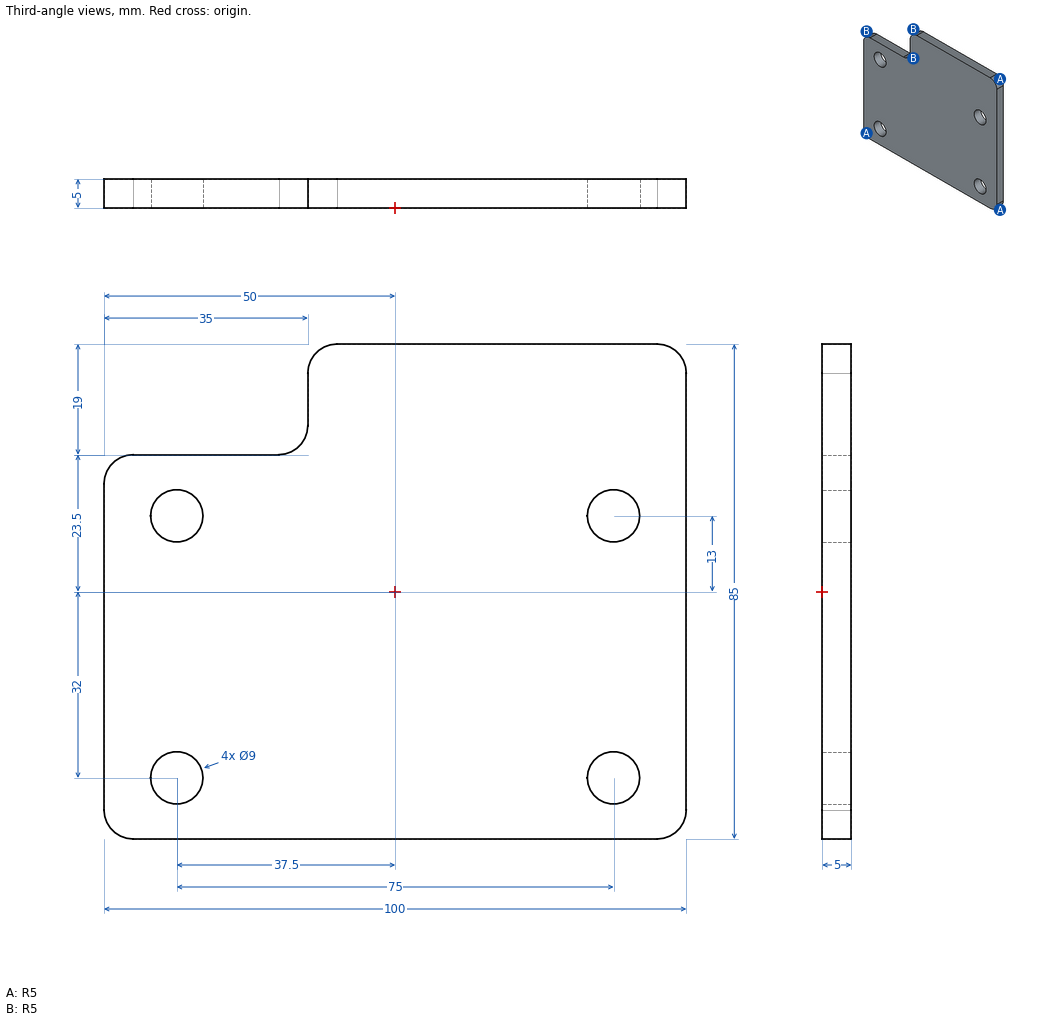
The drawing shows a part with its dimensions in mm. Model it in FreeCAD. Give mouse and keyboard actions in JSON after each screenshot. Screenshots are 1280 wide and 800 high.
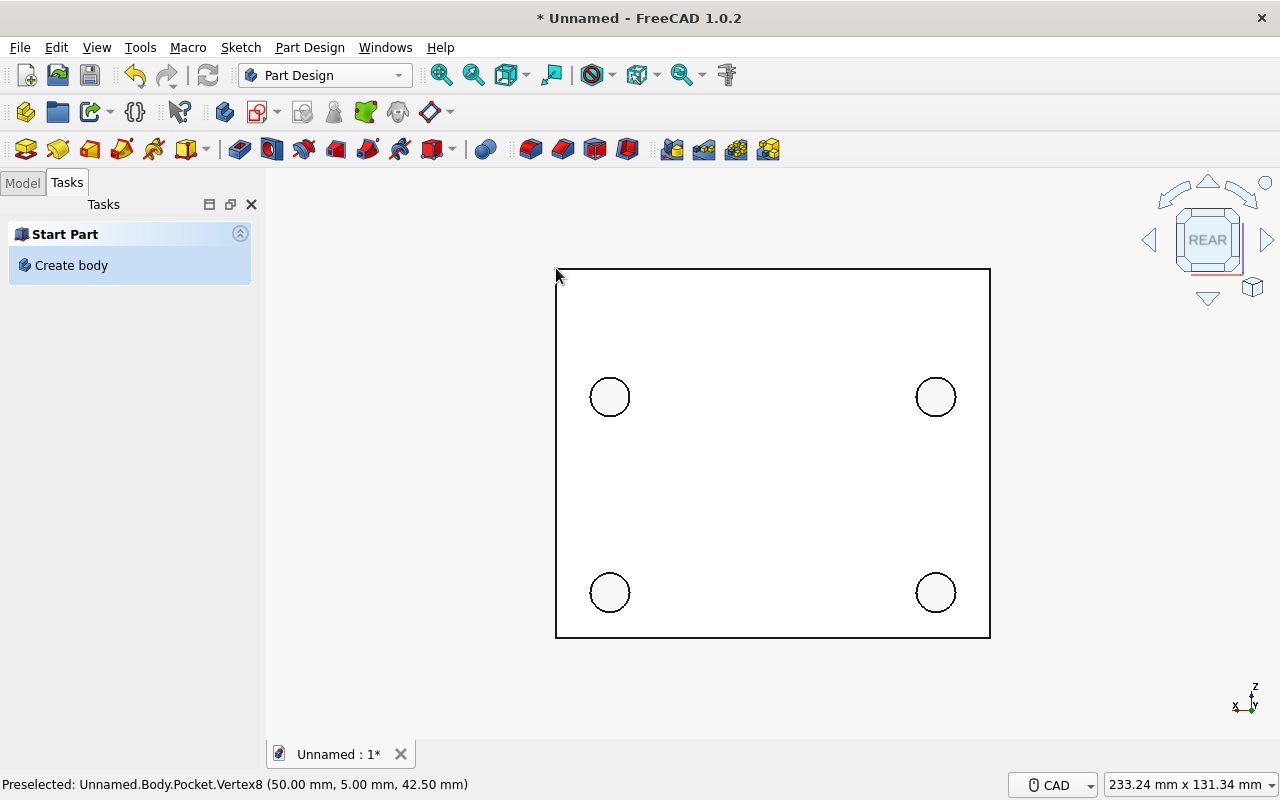
{"action": "key", "text": "0"}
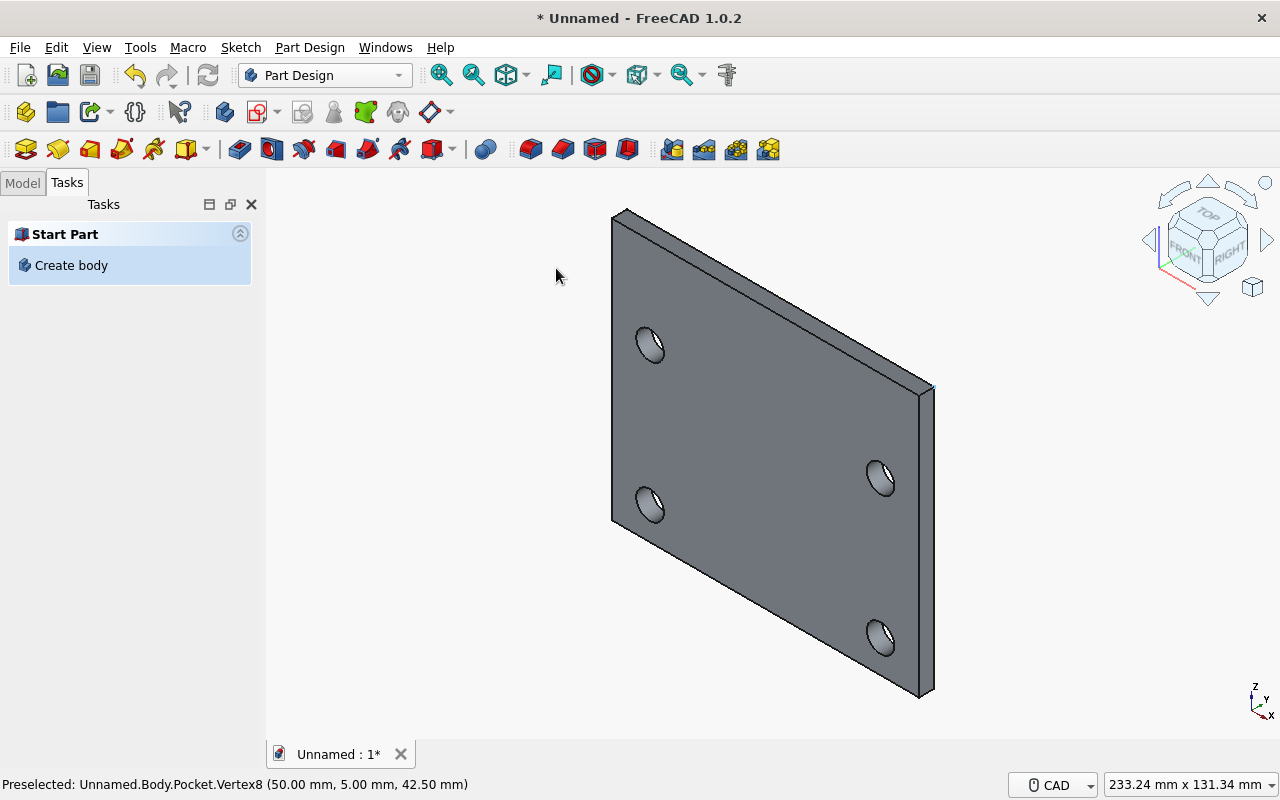
{"action": "left_click", "coordinate": [927, 390]}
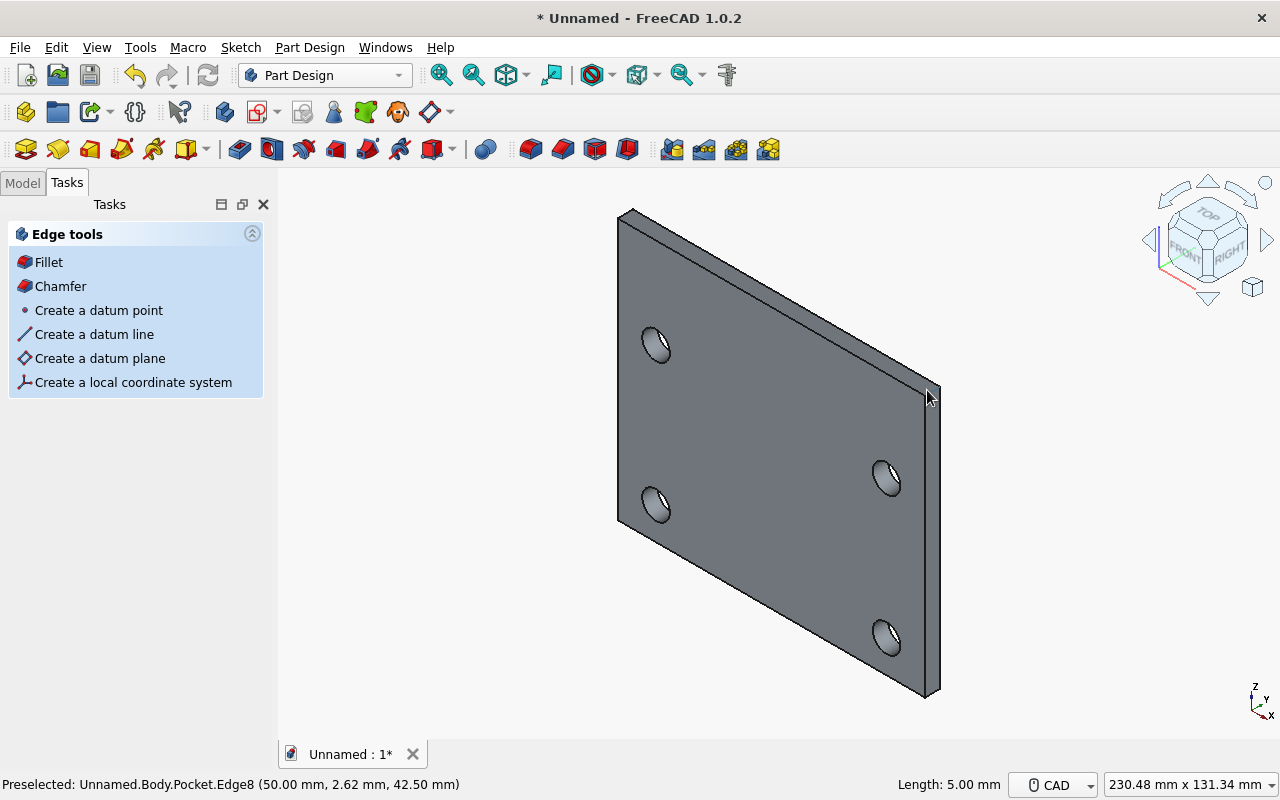
{"action": "scroll", "coordinate": [625, 515], "scroll_direction": "up", "scroll_amount": 4}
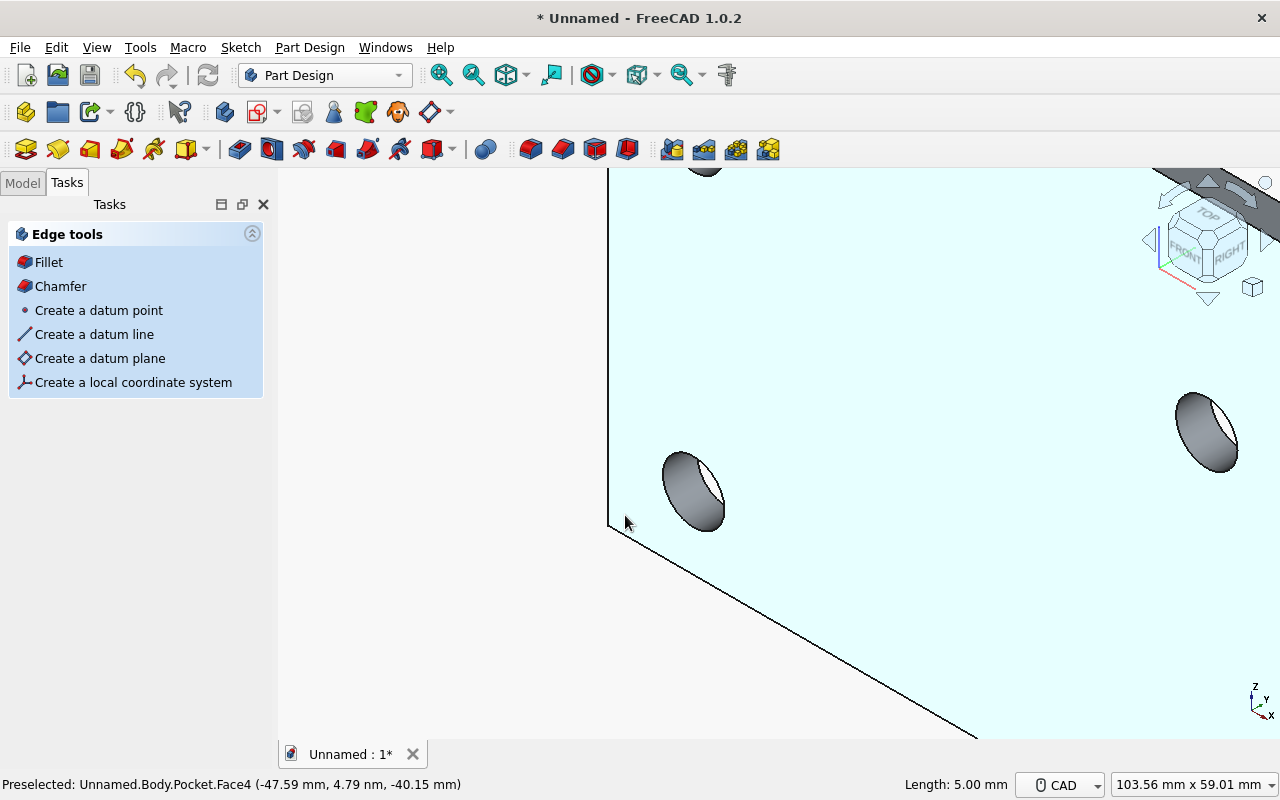
{"action": "left_click", "coordinate": [442, 76]}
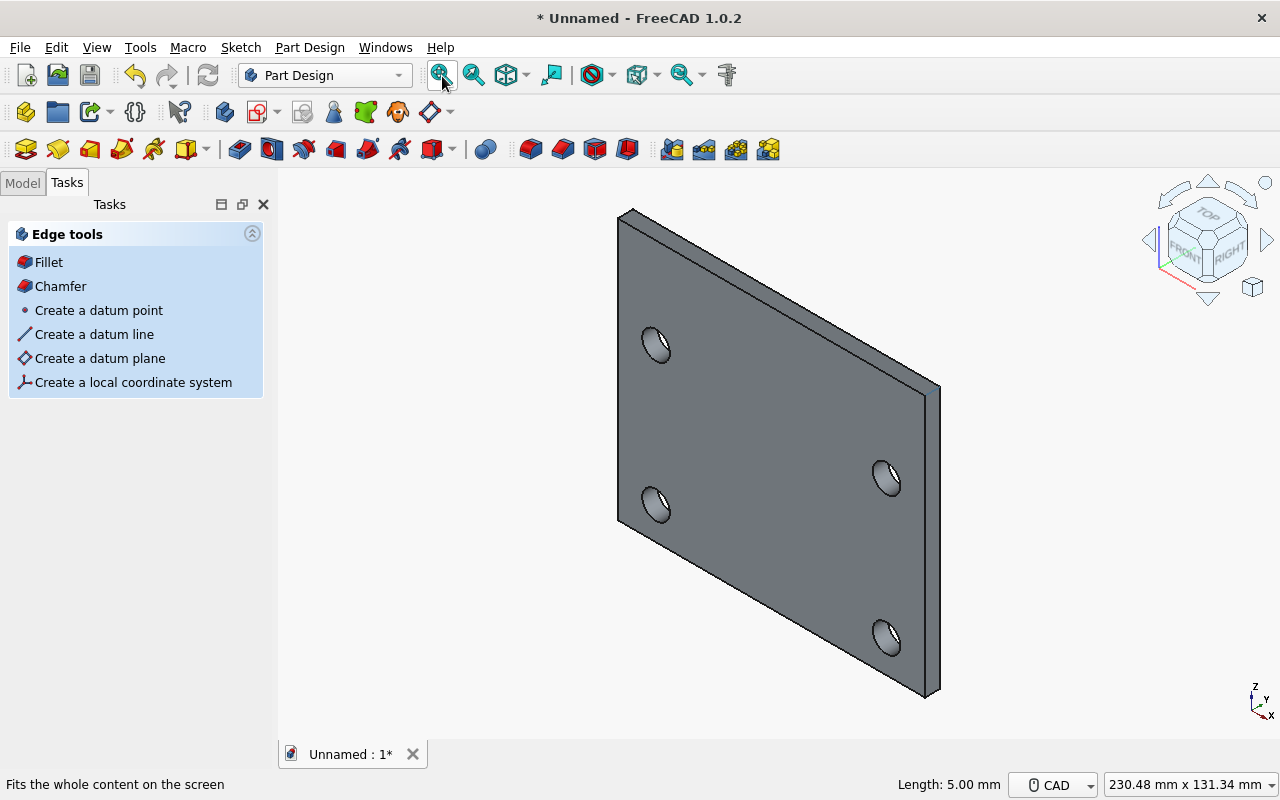
{"action": "key", "text": "2"}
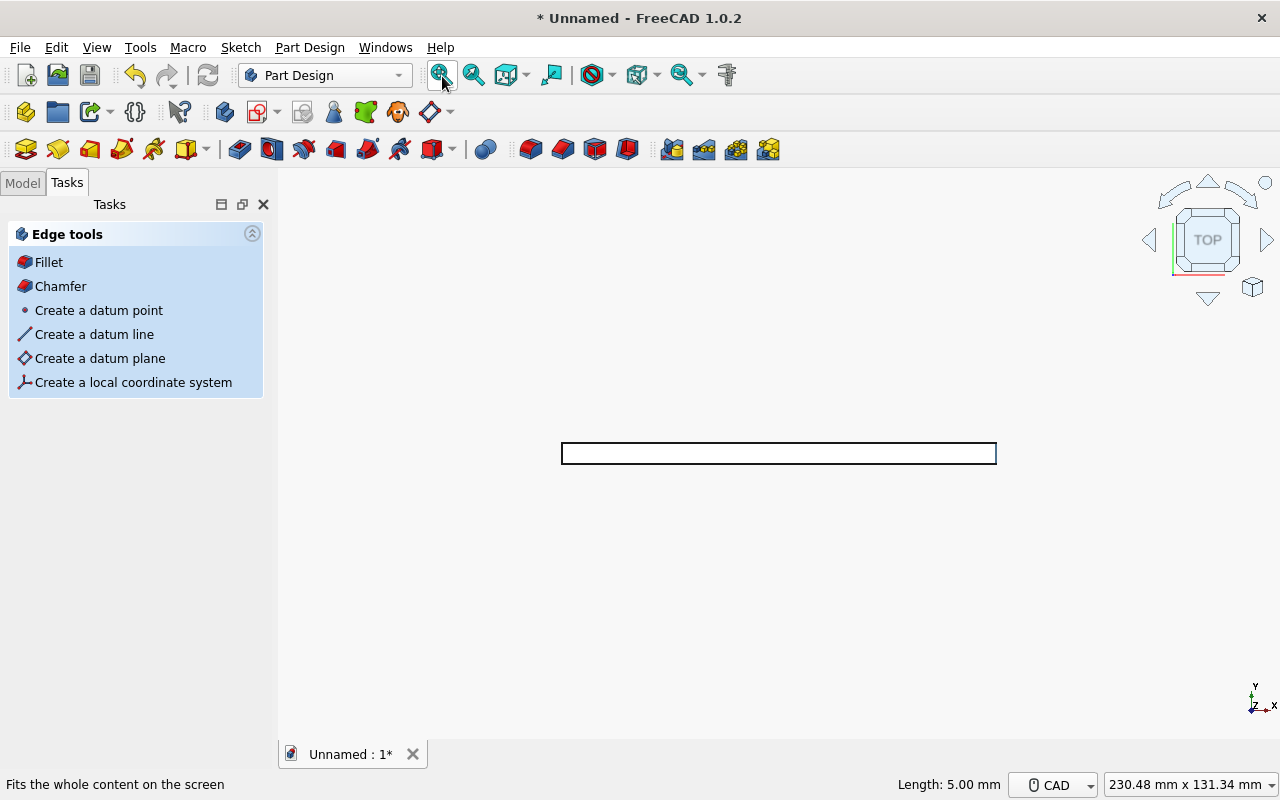
{"action": "left_click", "coordinate": [442, 76]}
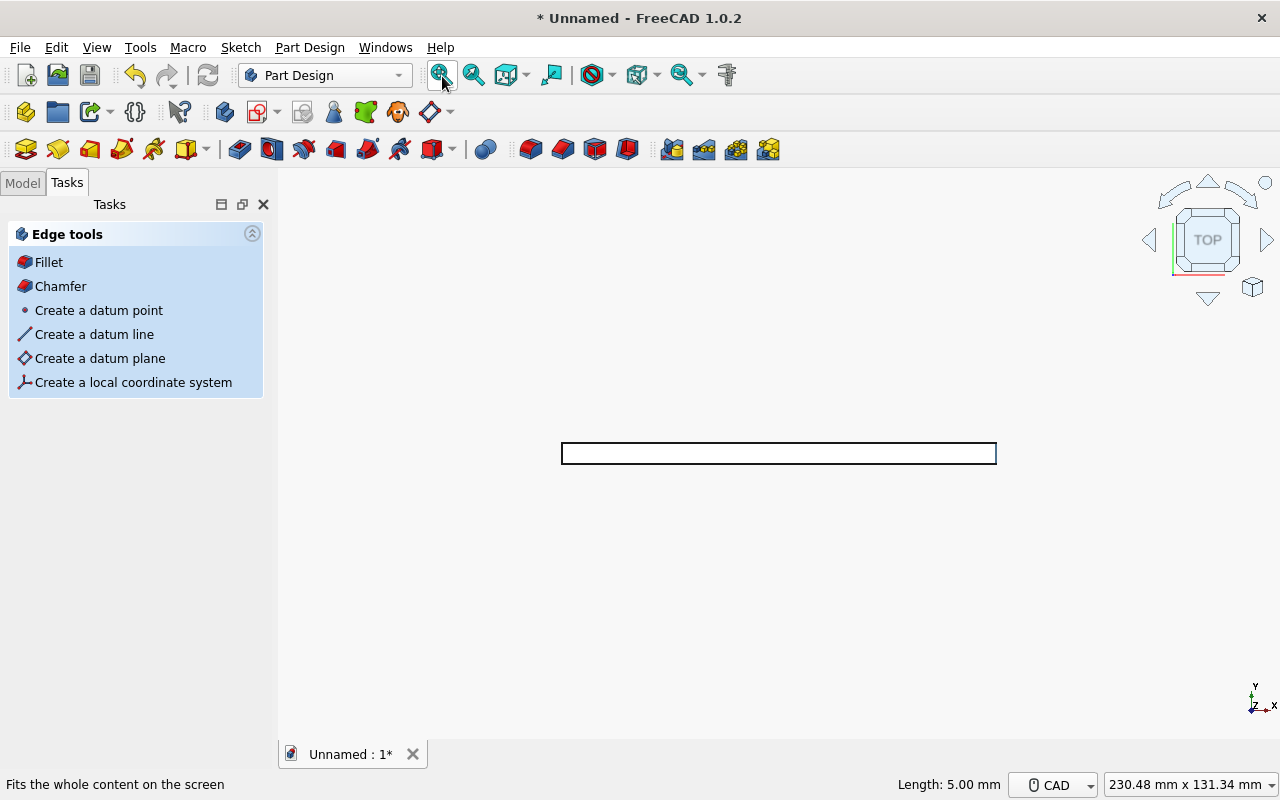
{"action": "scroll", "coordinate": [562, 452], "scroll_direction": "up", "scroll_amount": 4}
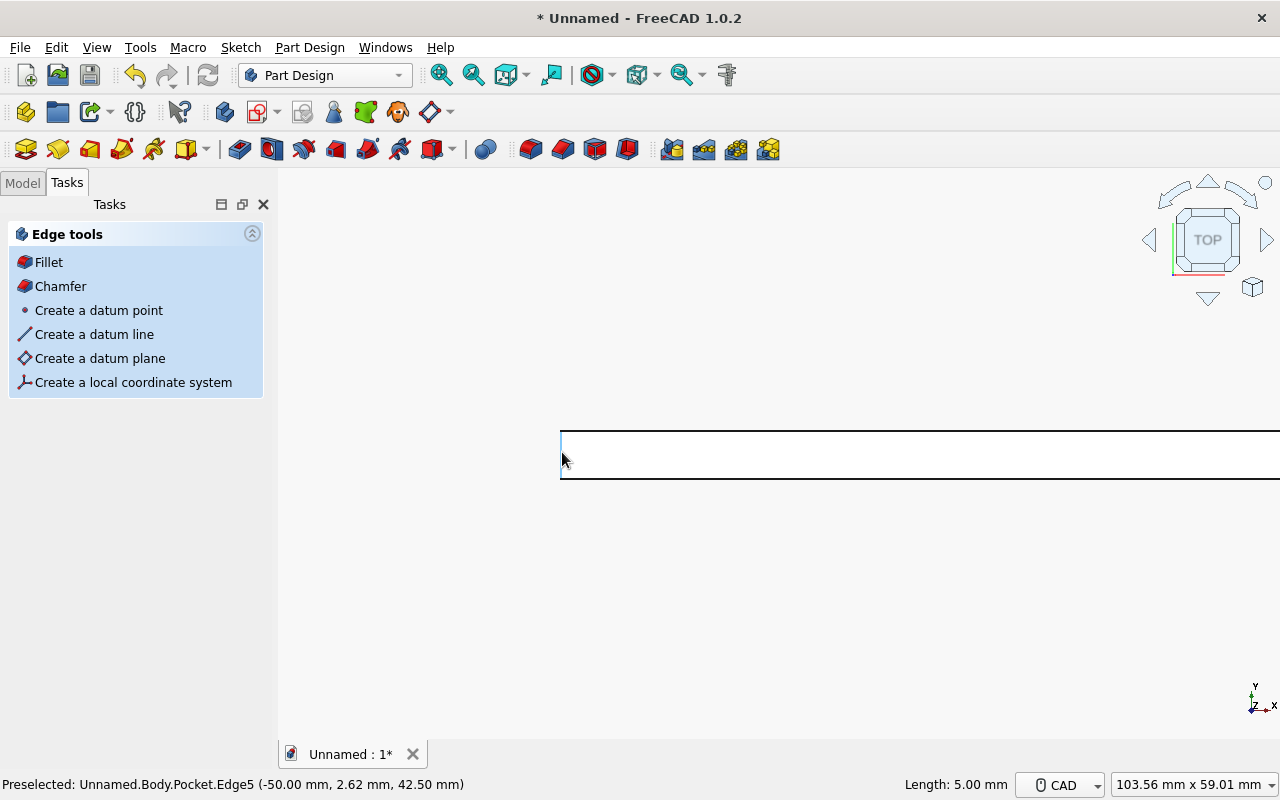
{"action": "left_click", "coordinate": [442, 76]}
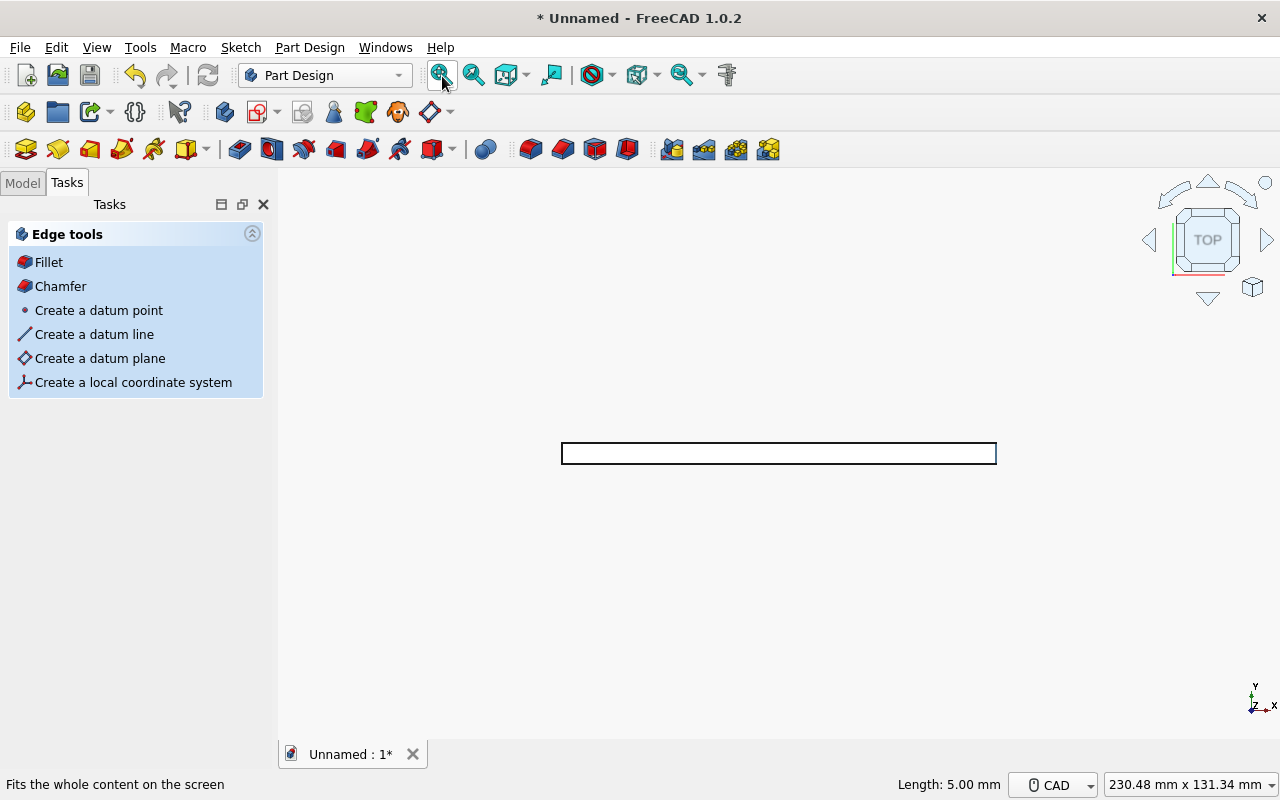
{"action": "key", "text": "1"}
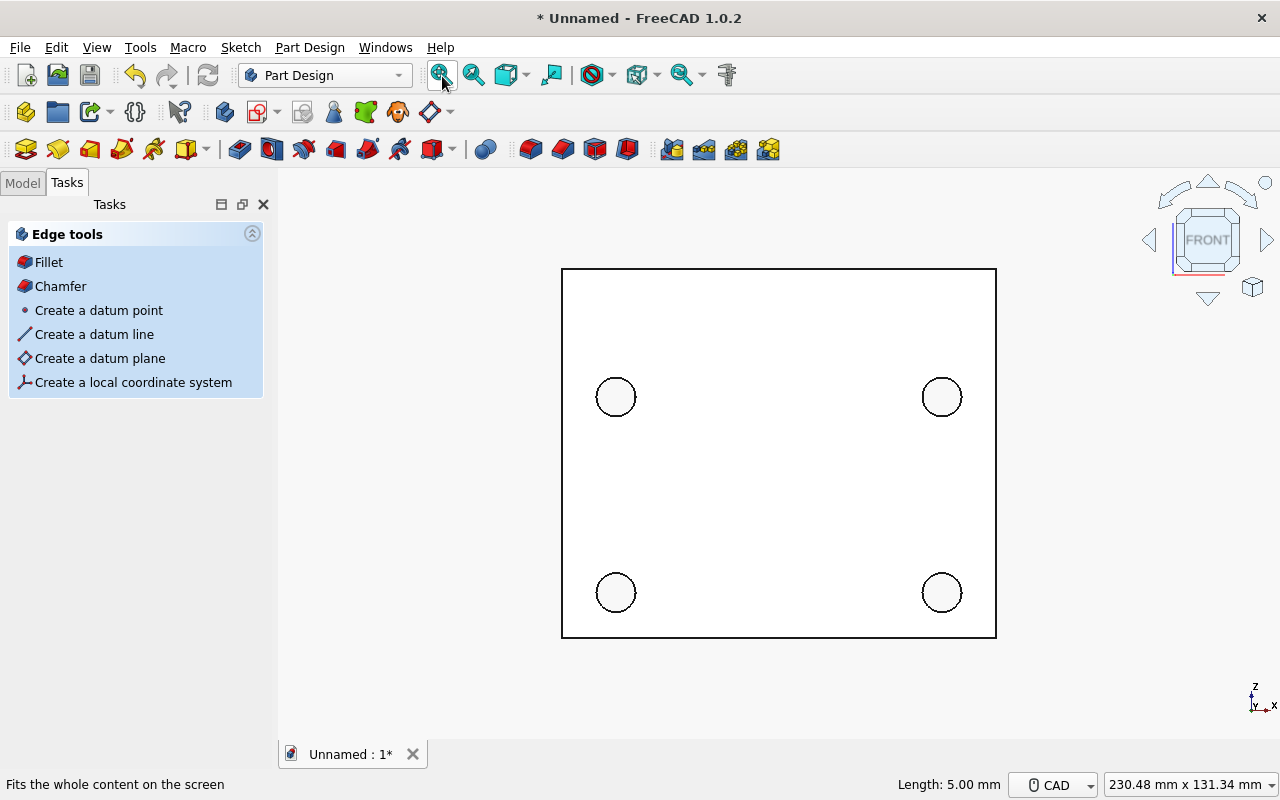
{"action": "scroll", "coordinate": [562, 637], "scroll_direction": "up", "scroll_amount": 4}